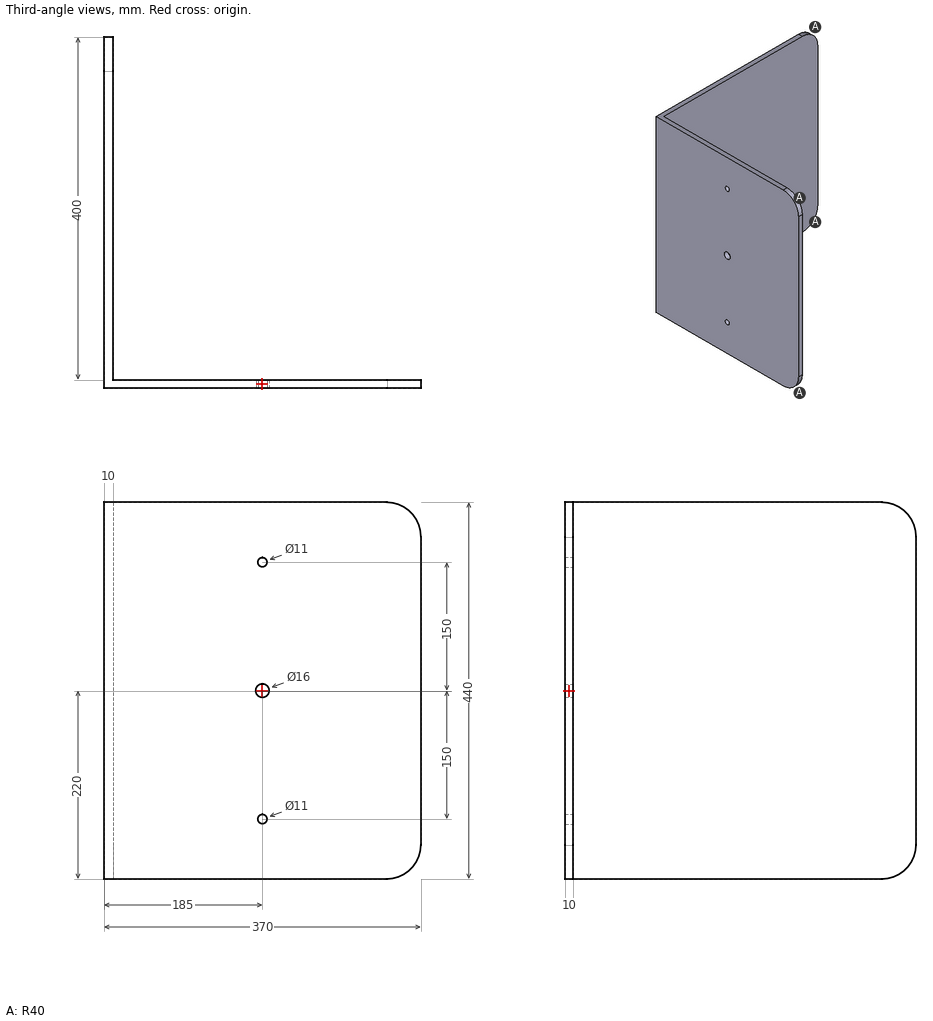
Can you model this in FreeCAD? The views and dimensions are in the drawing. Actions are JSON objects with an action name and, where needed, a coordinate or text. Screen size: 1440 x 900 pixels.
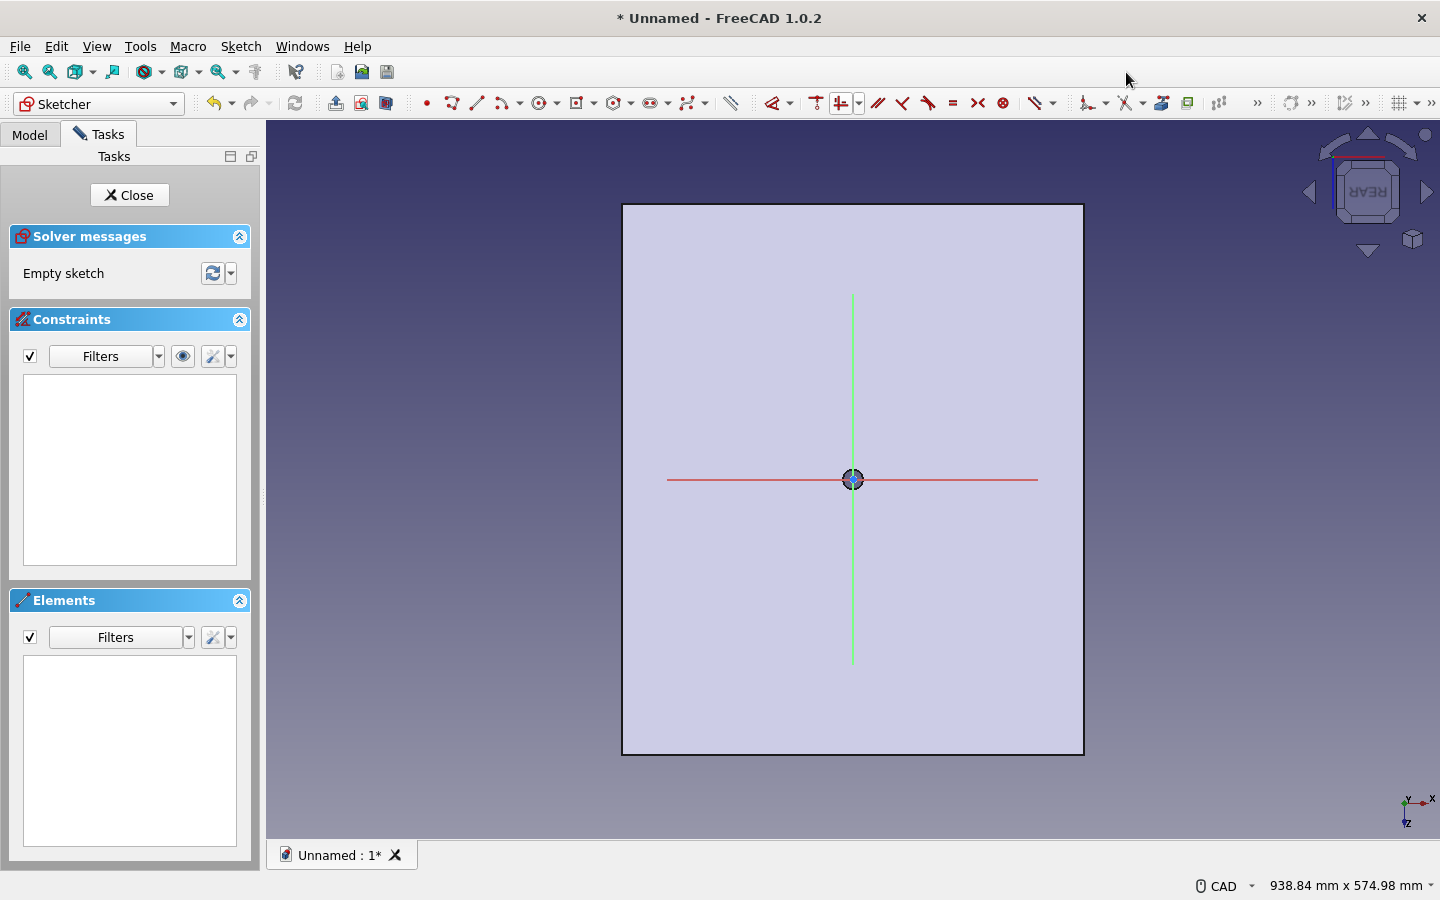
{"action": "scroll", "coordinate": [857, 282], "scroll_direction": "up", "scroll_amount": 15}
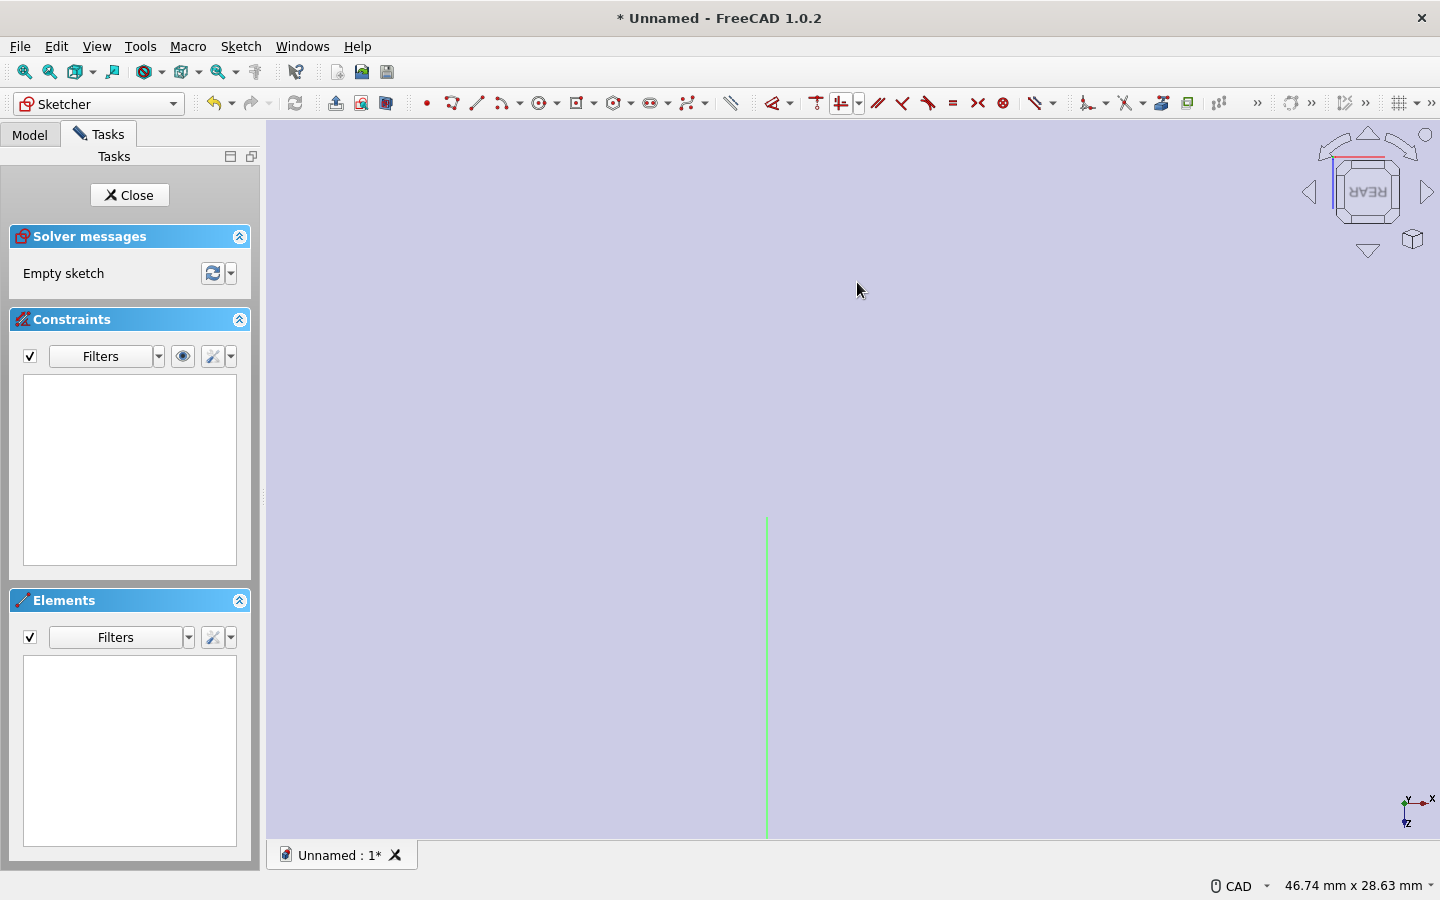
{"action": "scroll", "coordinate": [746, 474], "scroll_direction": "up", "scroll_amount": 3}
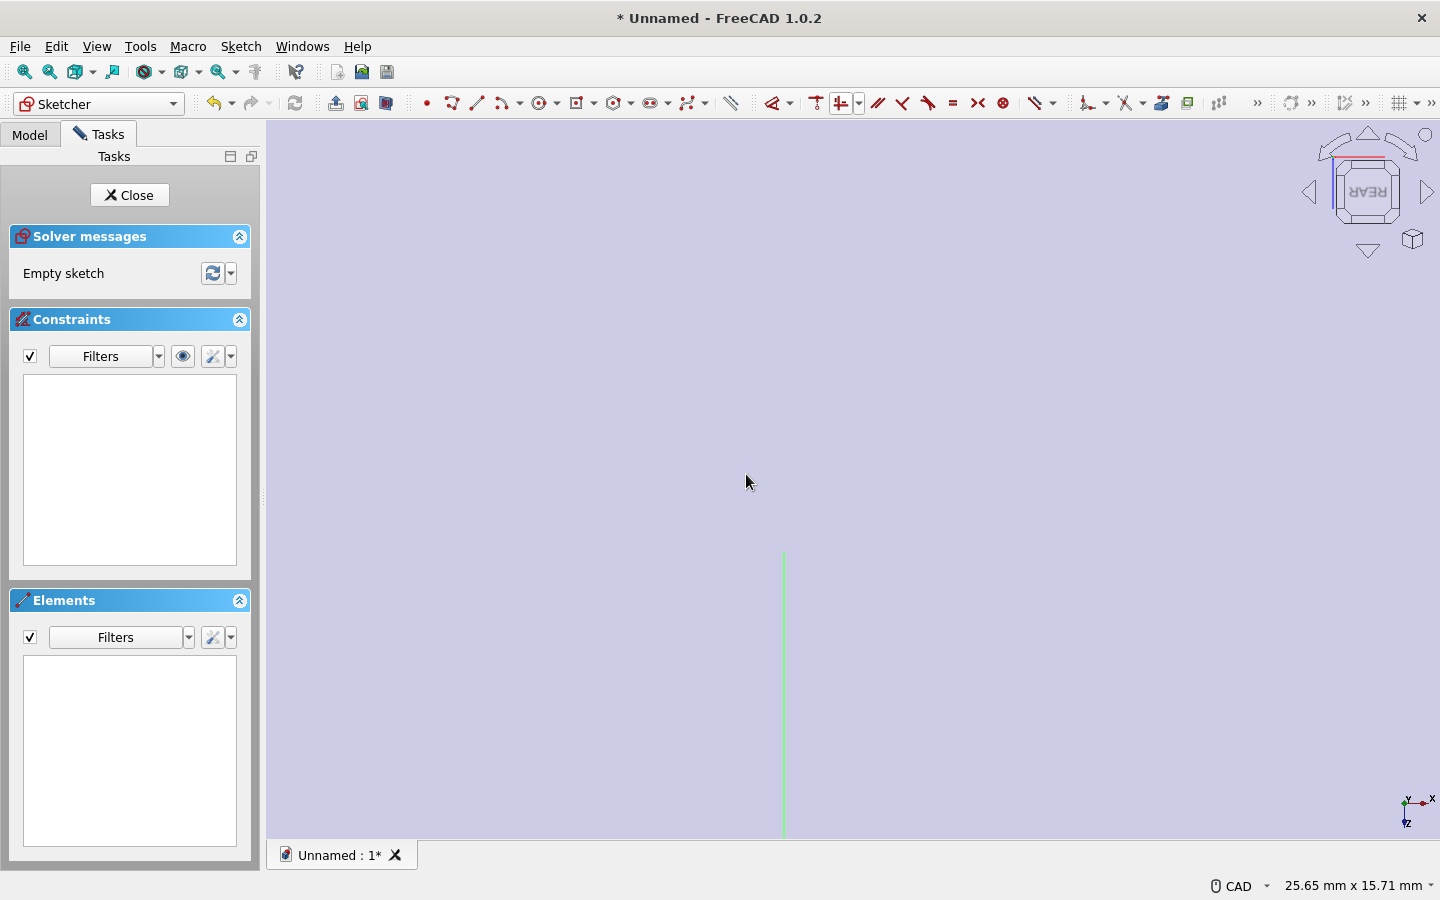
{"action": "left_click", "coordinate": [538, 104]}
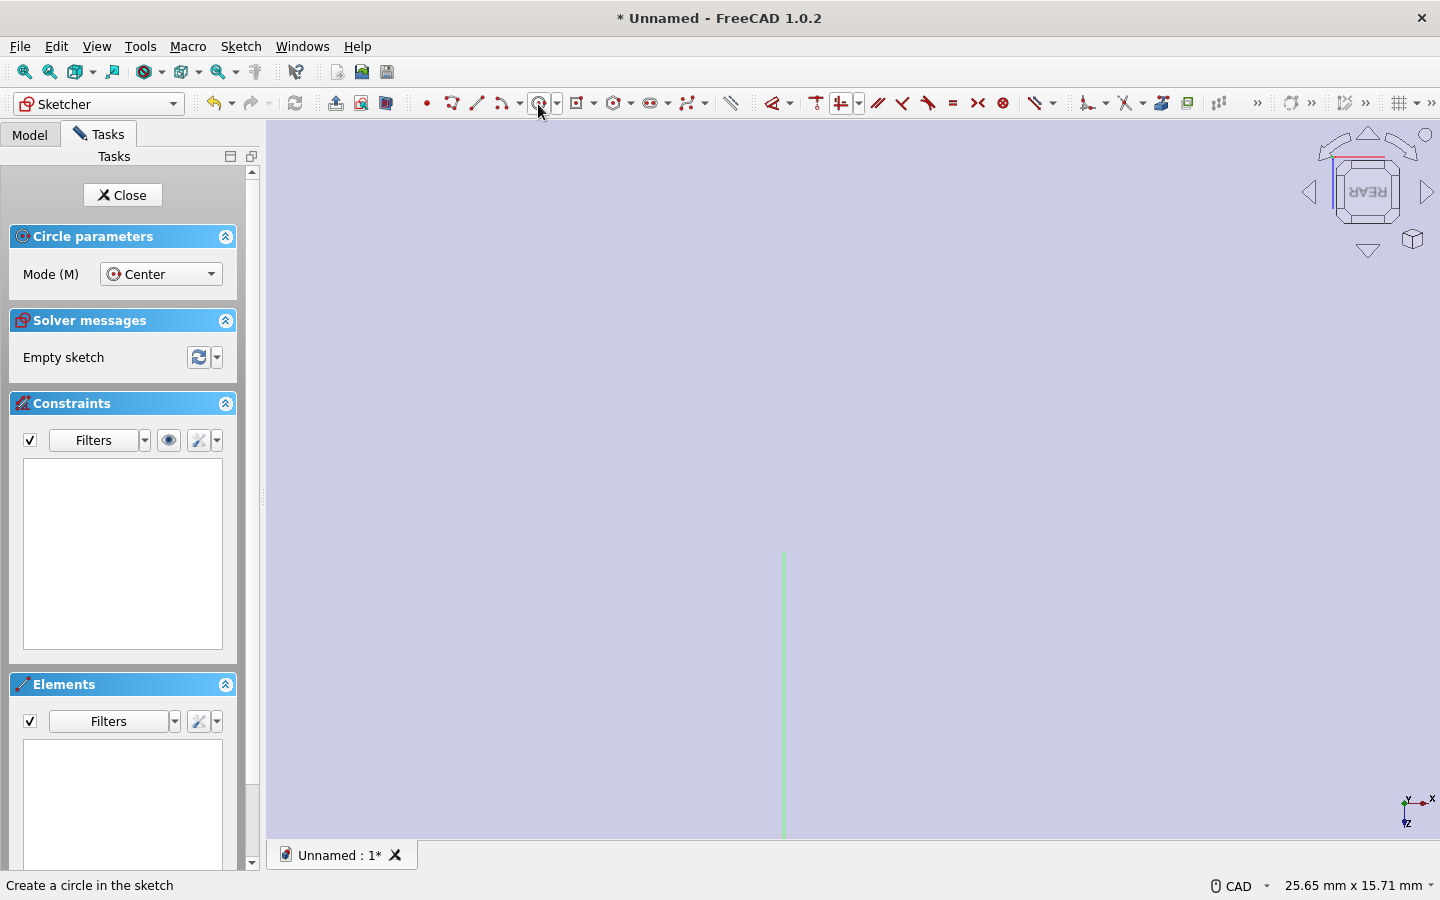
{"action": "left_click", "coordinate": [784, 479]}
{"action": "mouse_move", "coordinate": [962, 301]}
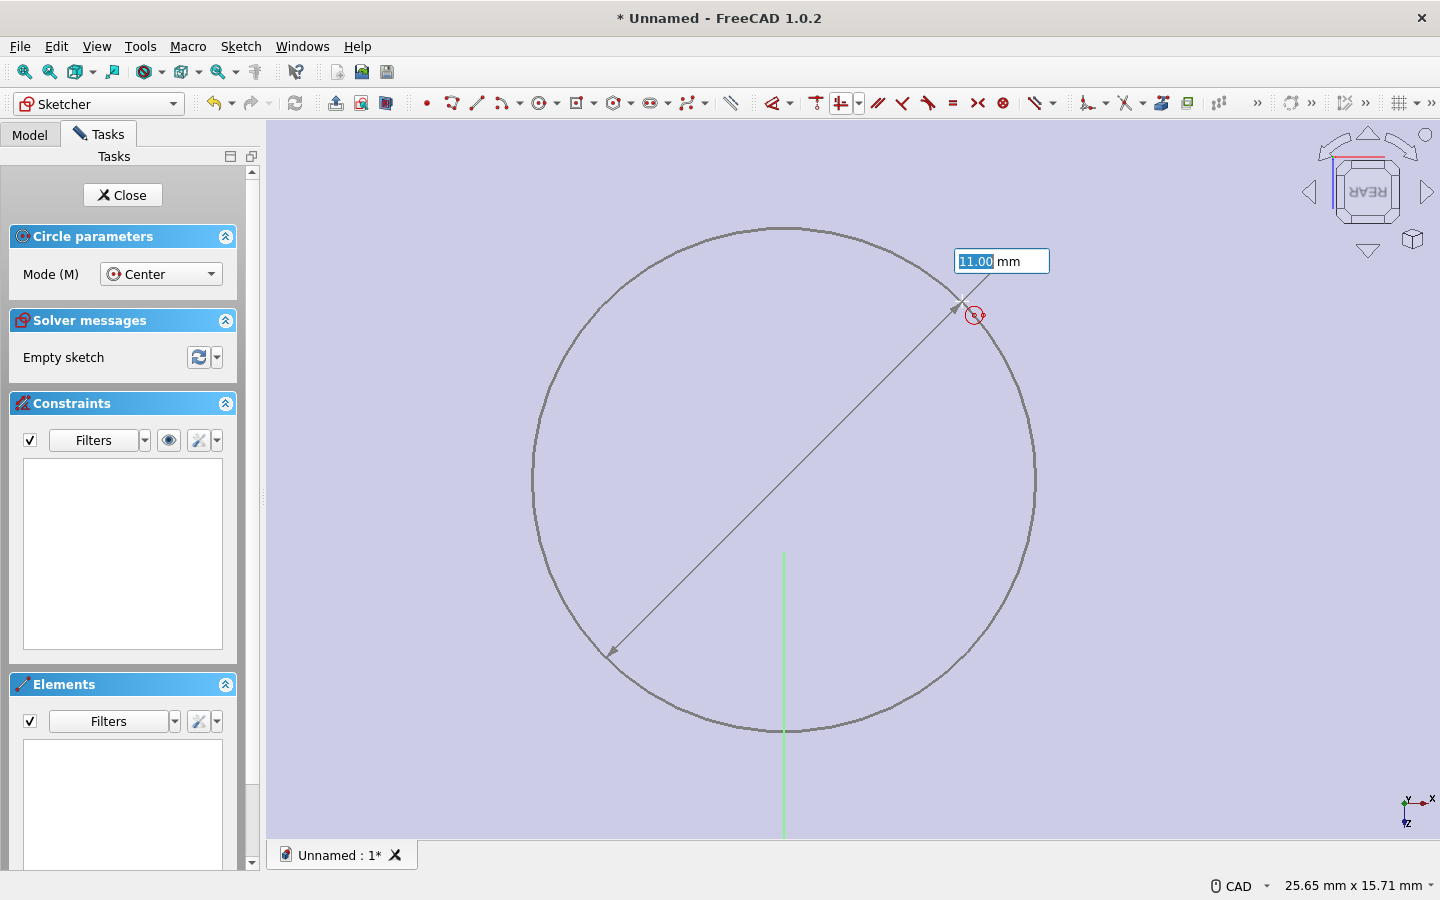
{"action": "type", "text": "11"}
{"action": "key", "text": "Return"}
{"action": "key", "text": "Escape"}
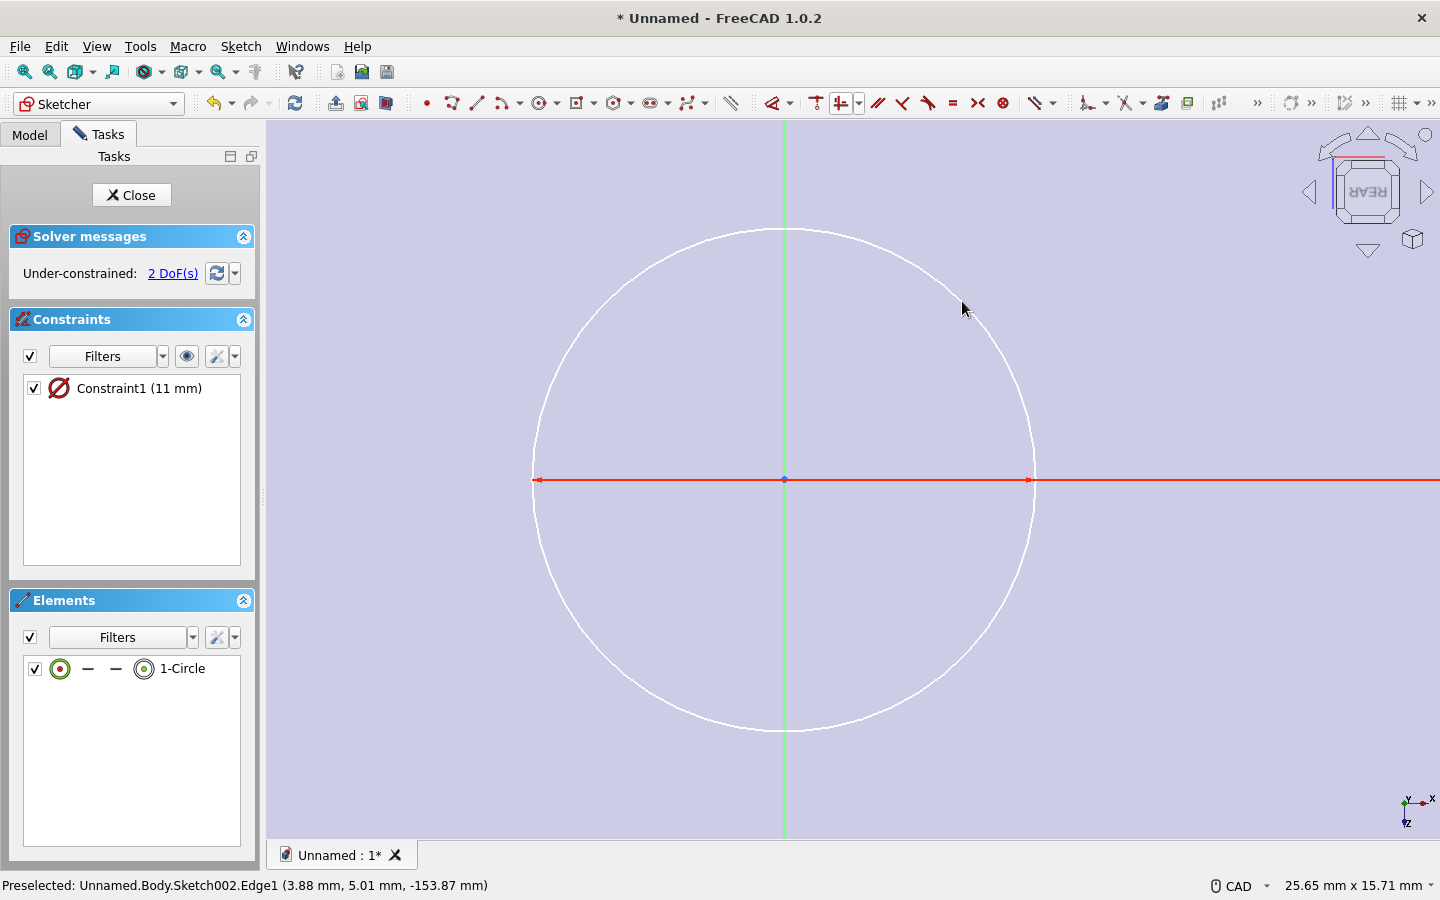
{"action": "left_click", "coordinate": [784, 480]}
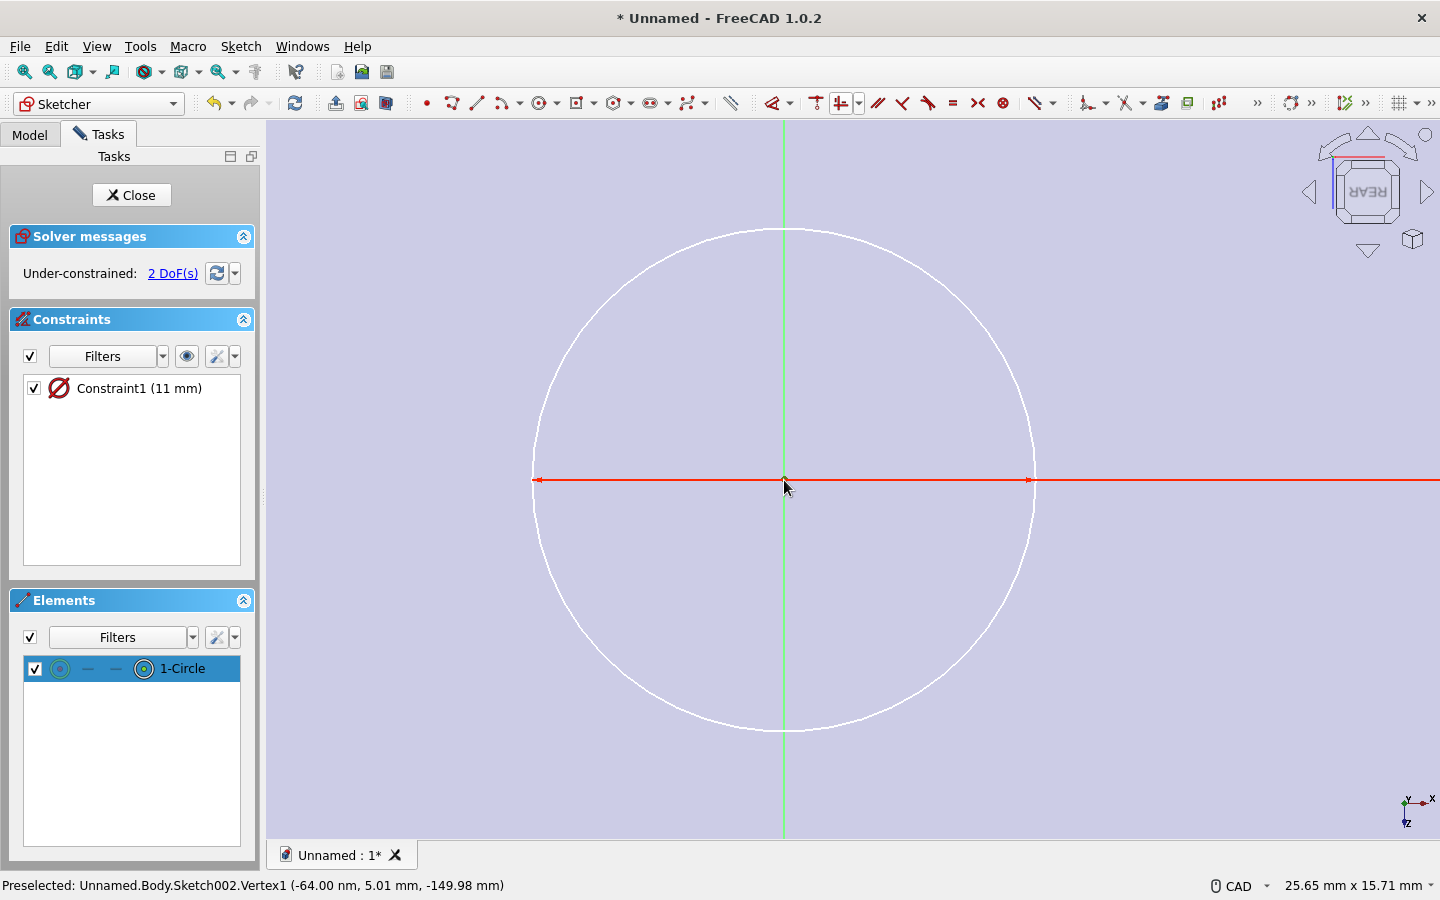
{"action": "left_click", "coordinate": [784, 764]}